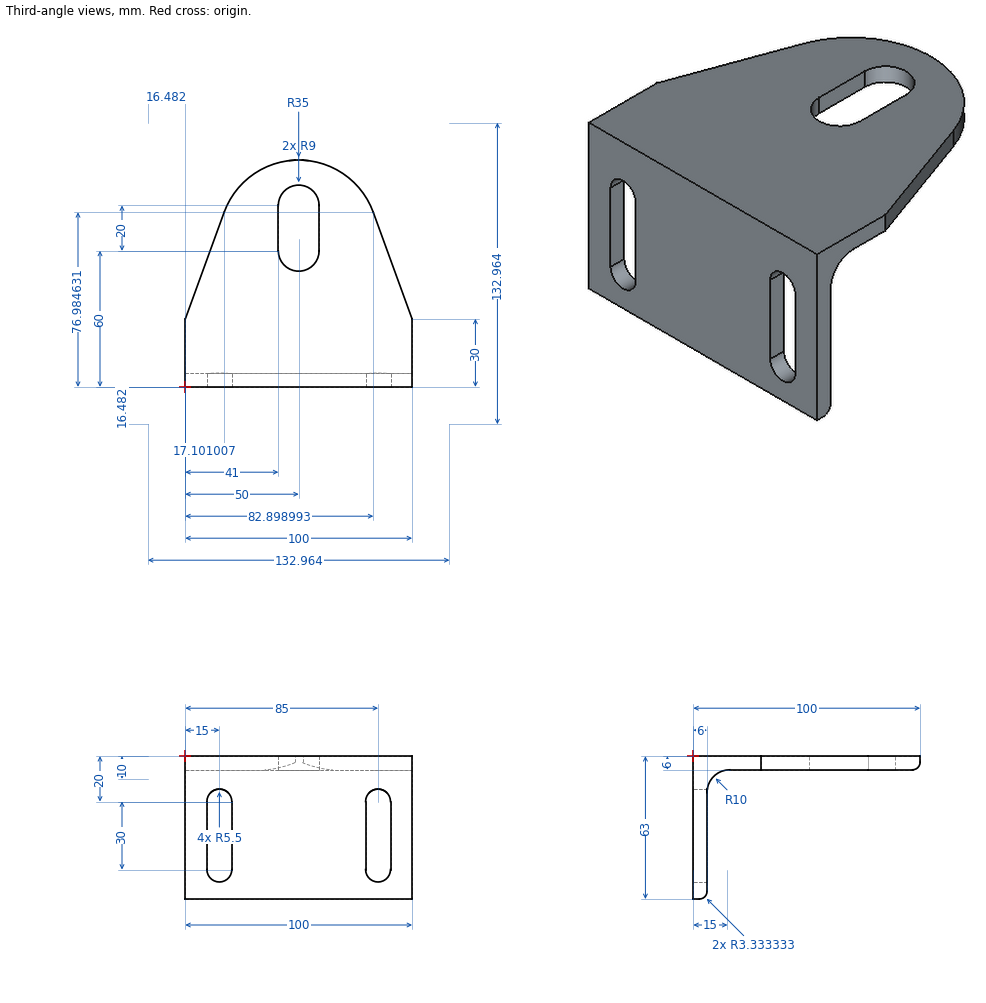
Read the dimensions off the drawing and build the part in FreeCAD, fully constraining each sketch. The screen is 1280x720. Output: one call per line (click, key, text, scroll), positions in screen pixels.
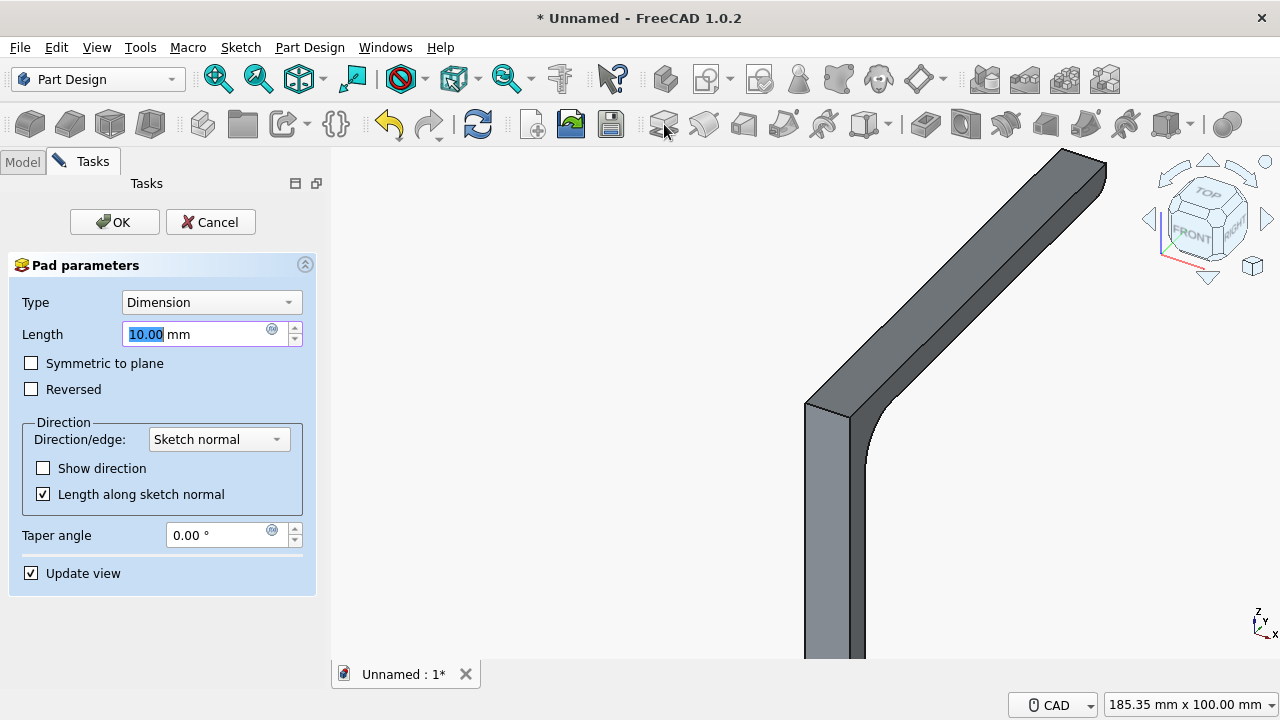
text(100)
key(Tab)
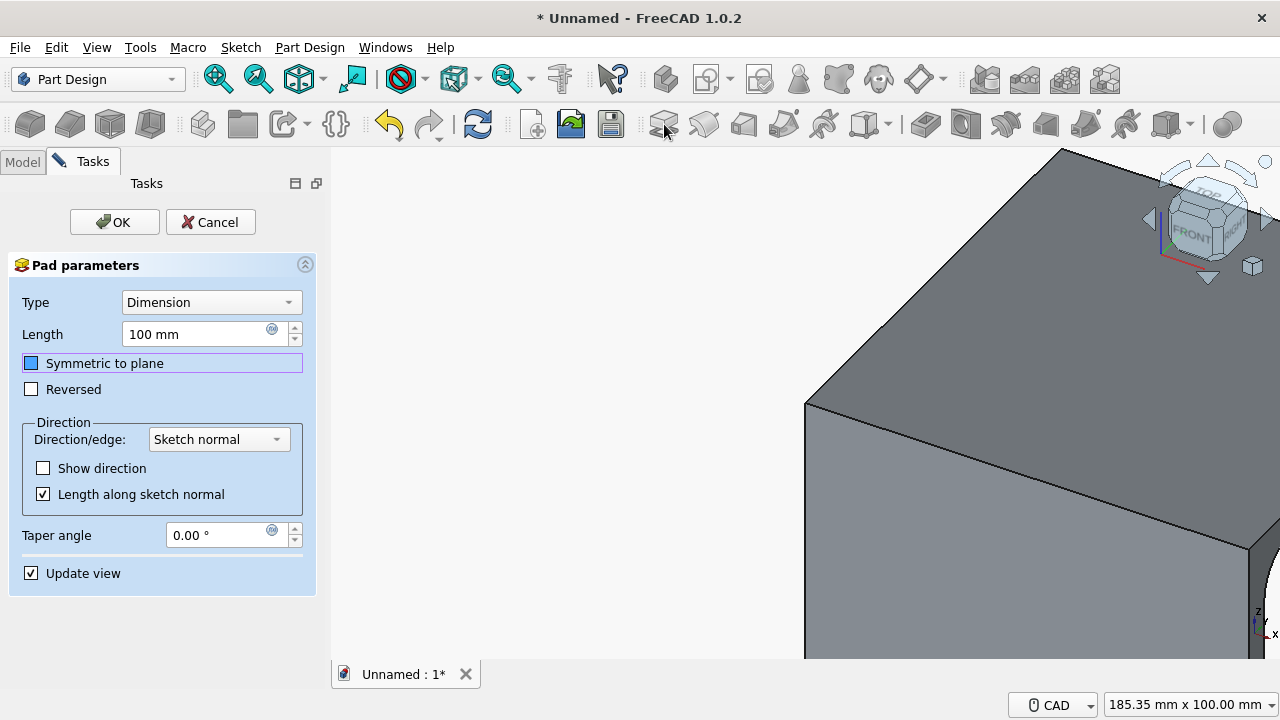
click(115, 222)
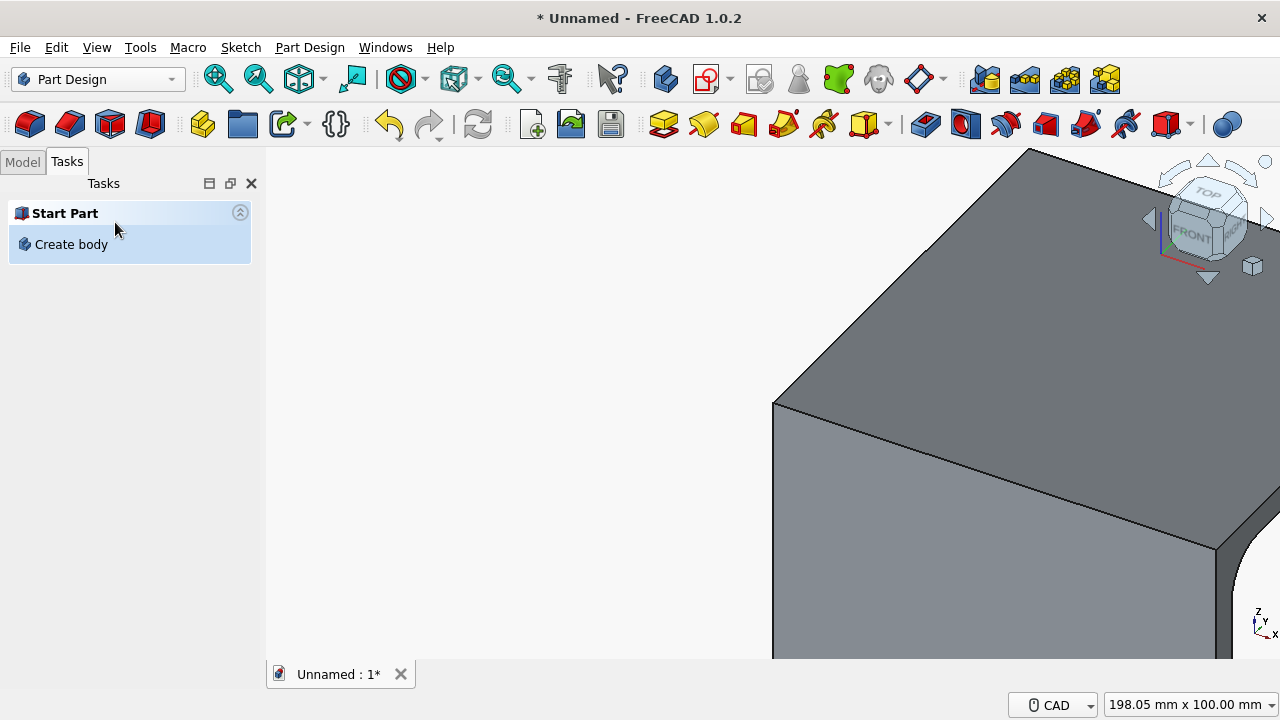
click(220, 80)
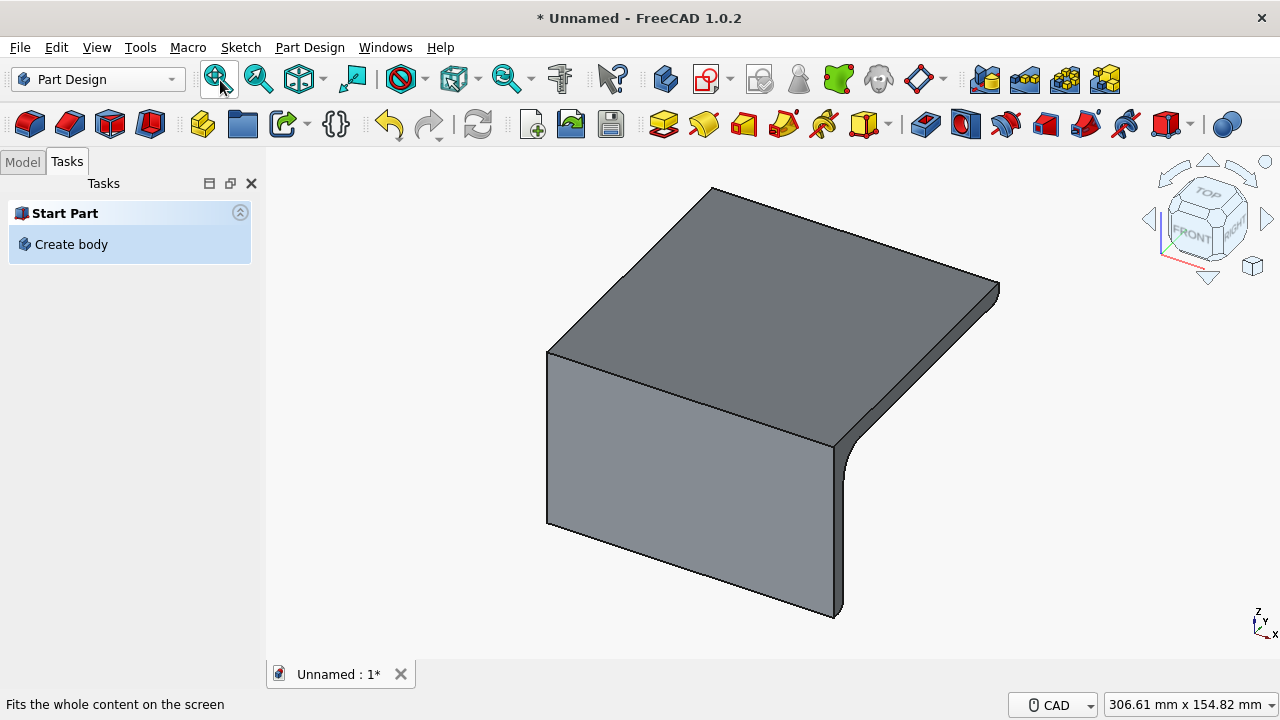
click(706, 80)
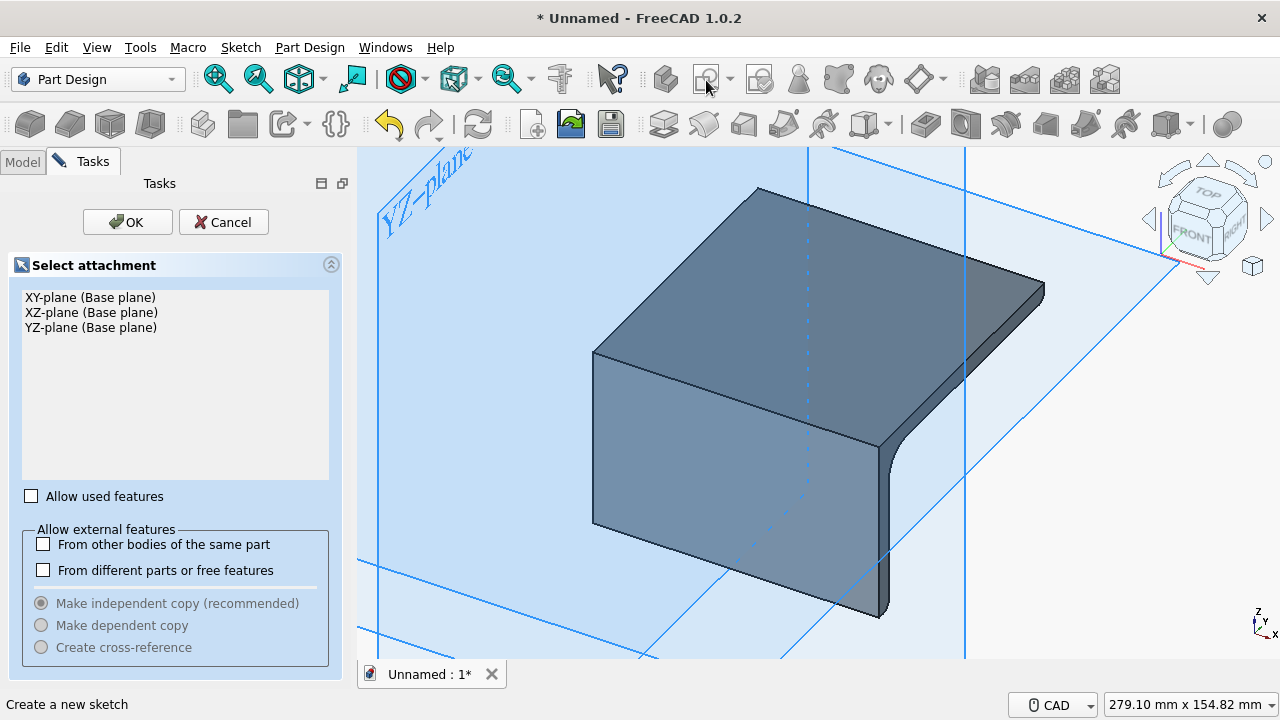
click(82, 298)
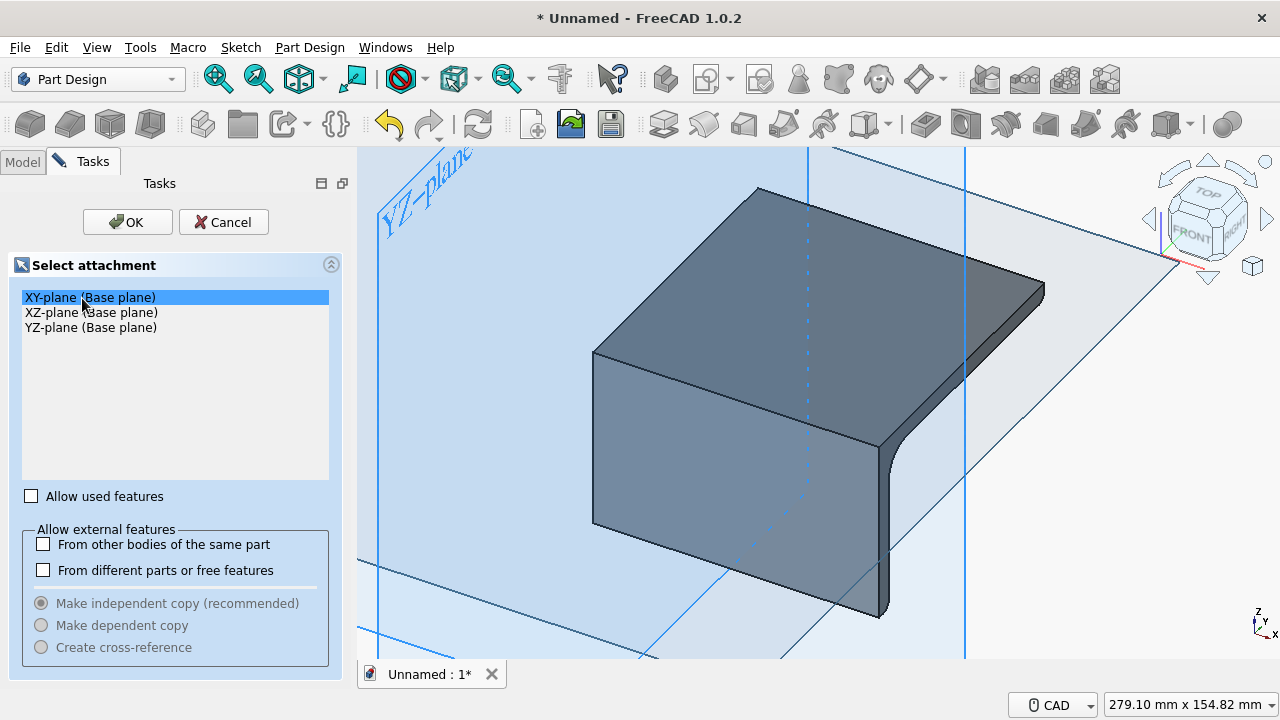
click(128, 222)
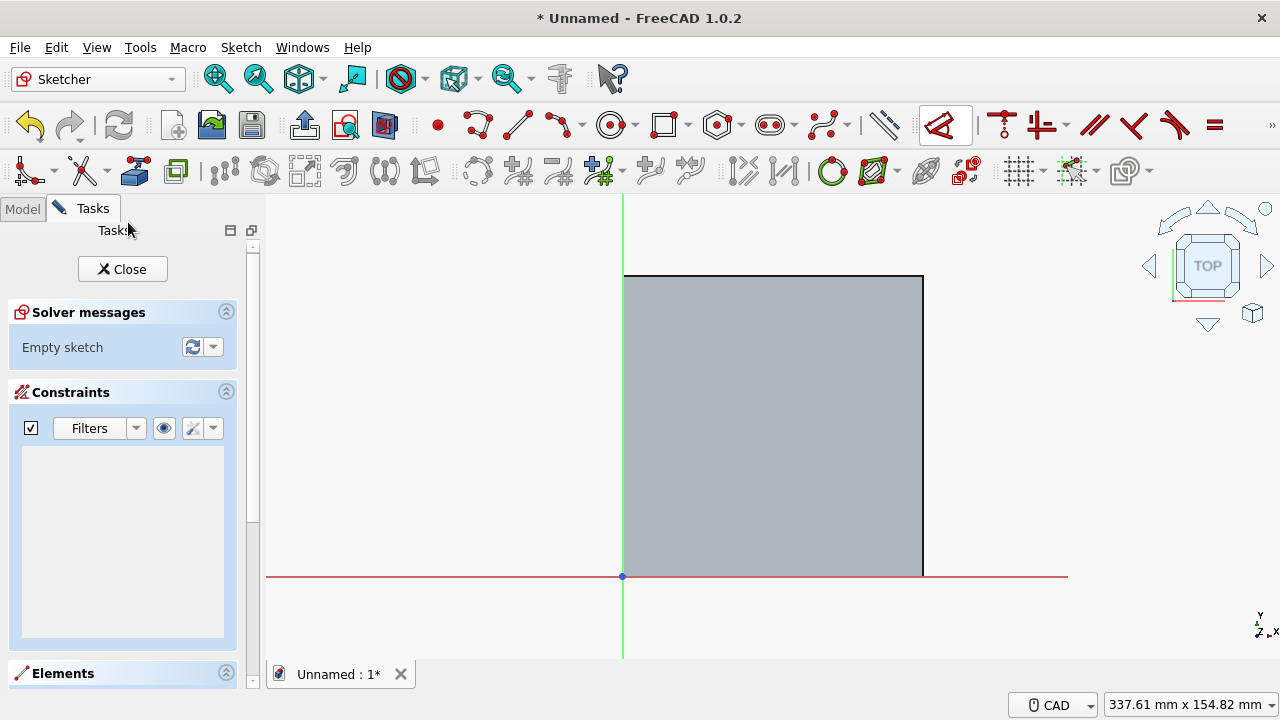
scroll(565, 427, down, 2)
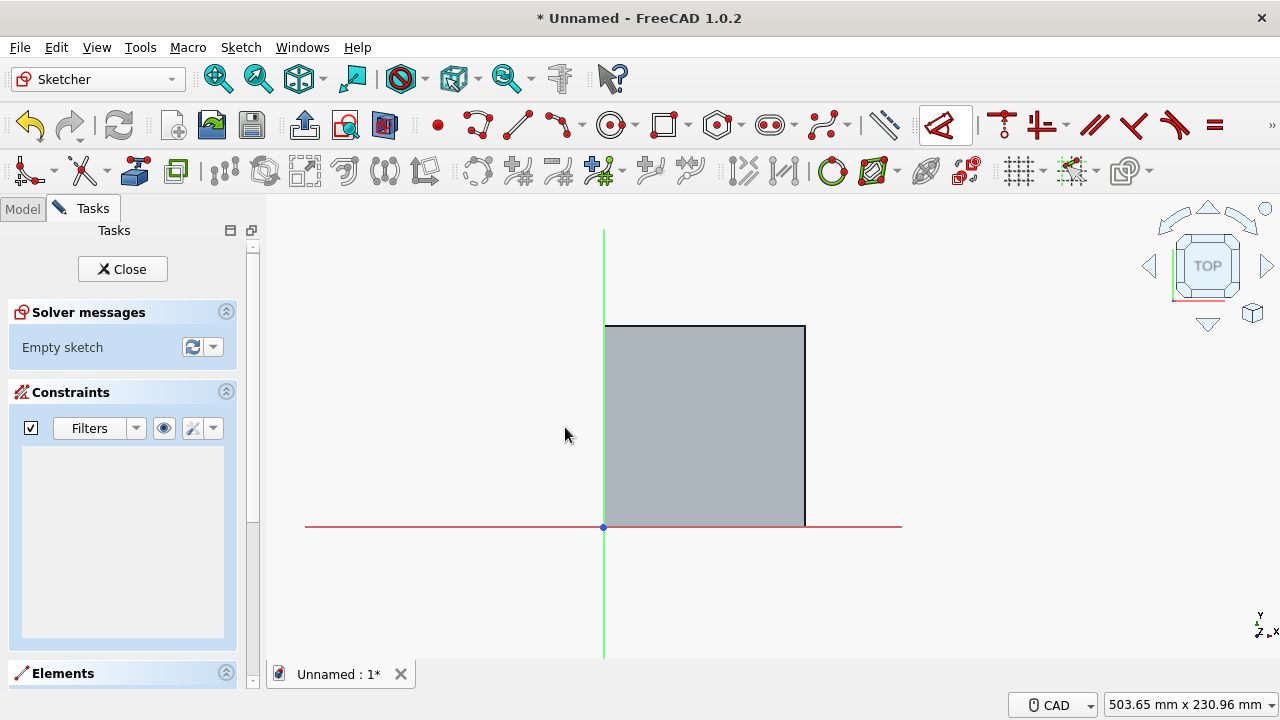
click(664, 126)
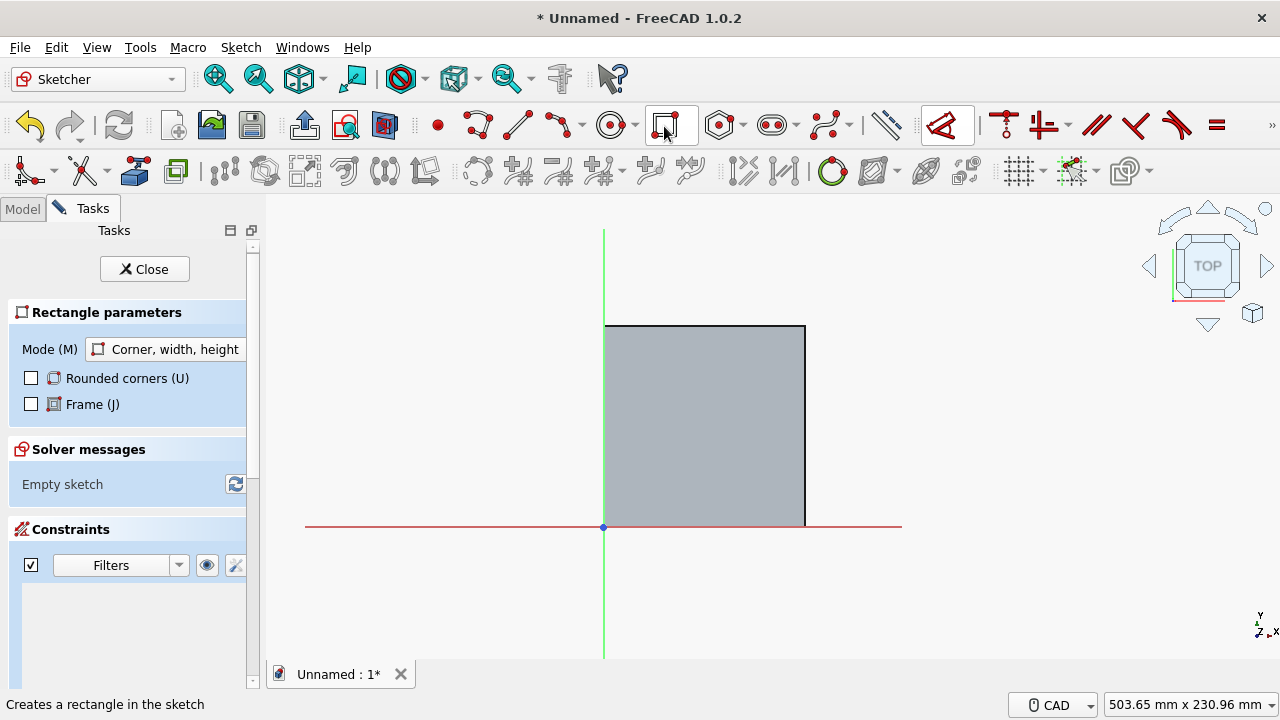
click(571, 293)
move(838, 561)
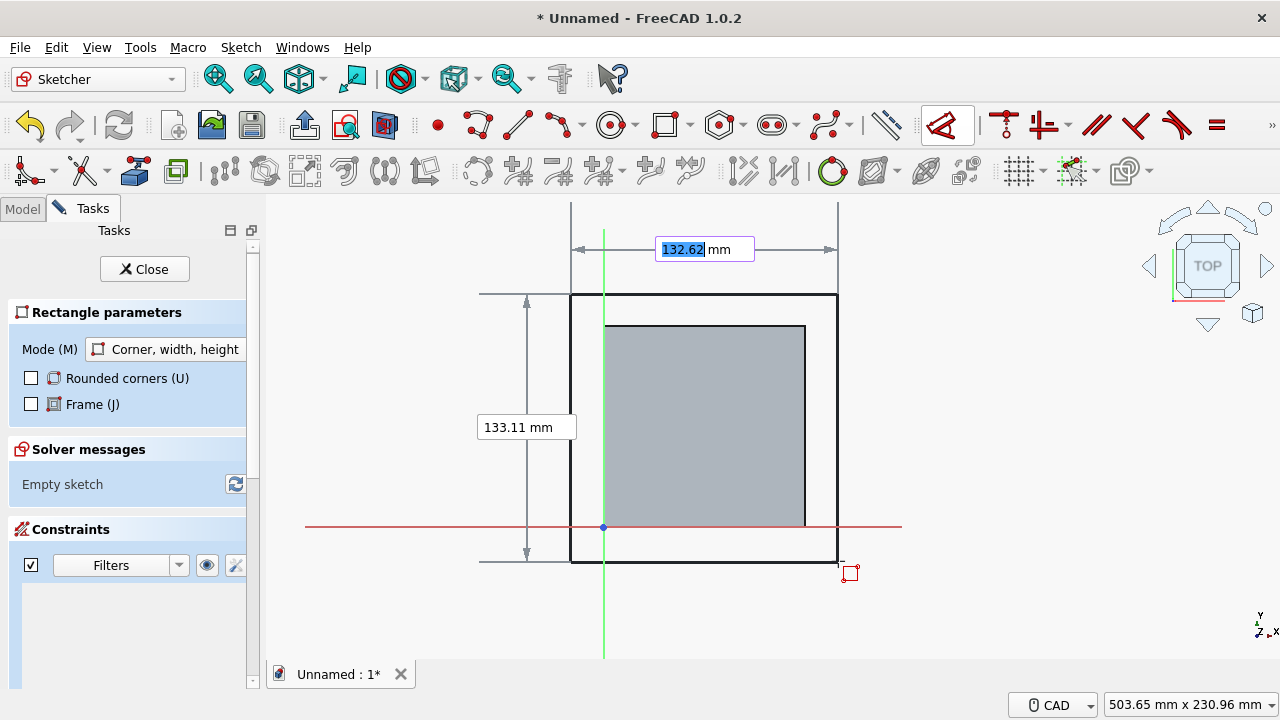
text(132.964)
key(Tab)
text(132.964)
key(Return)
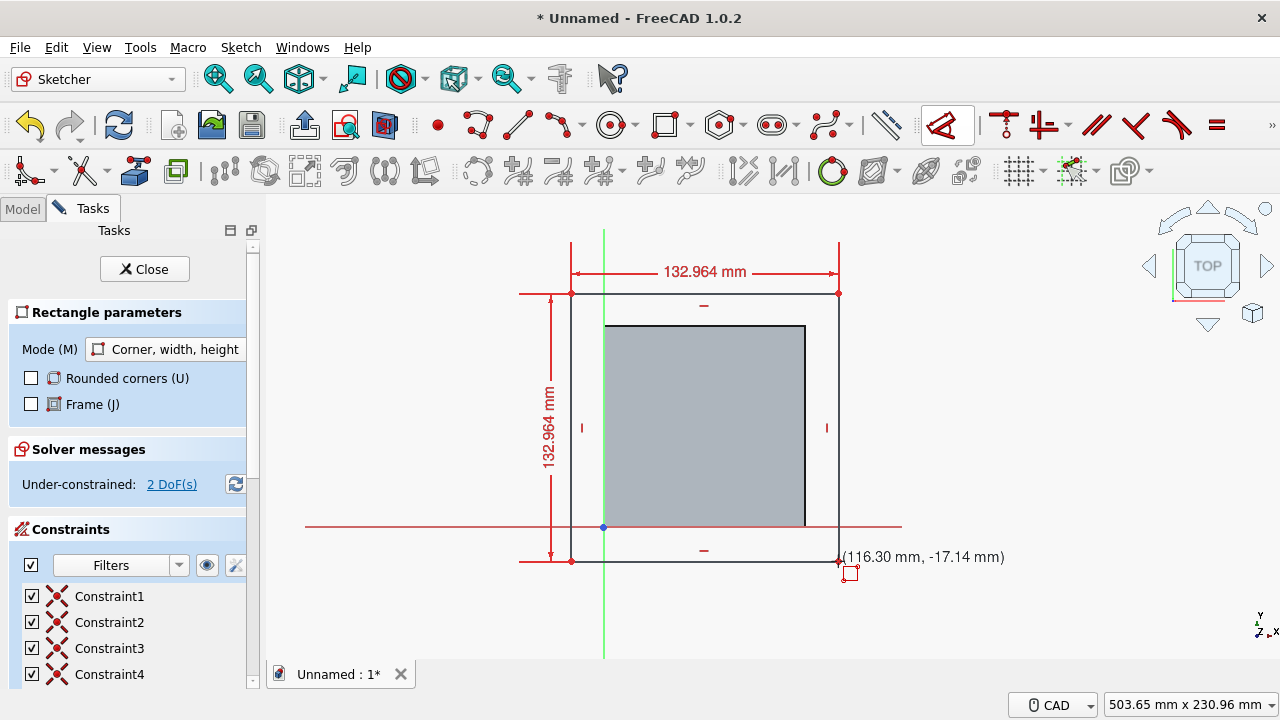
click(772, 126)